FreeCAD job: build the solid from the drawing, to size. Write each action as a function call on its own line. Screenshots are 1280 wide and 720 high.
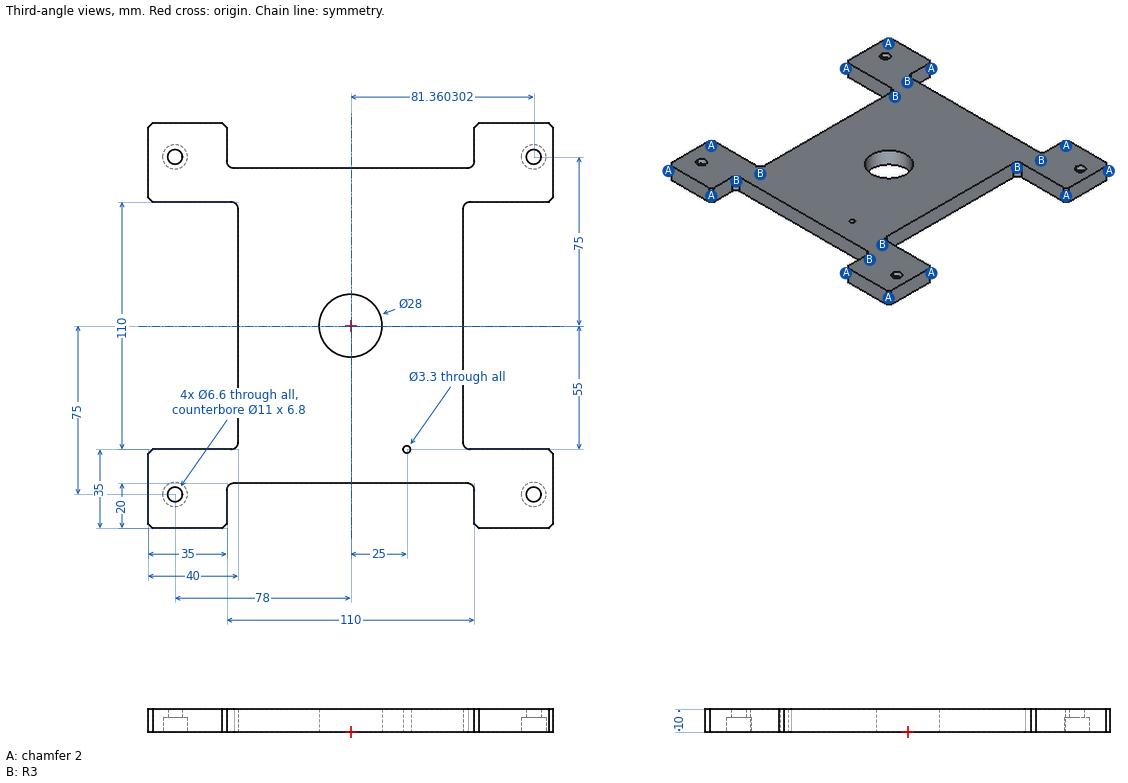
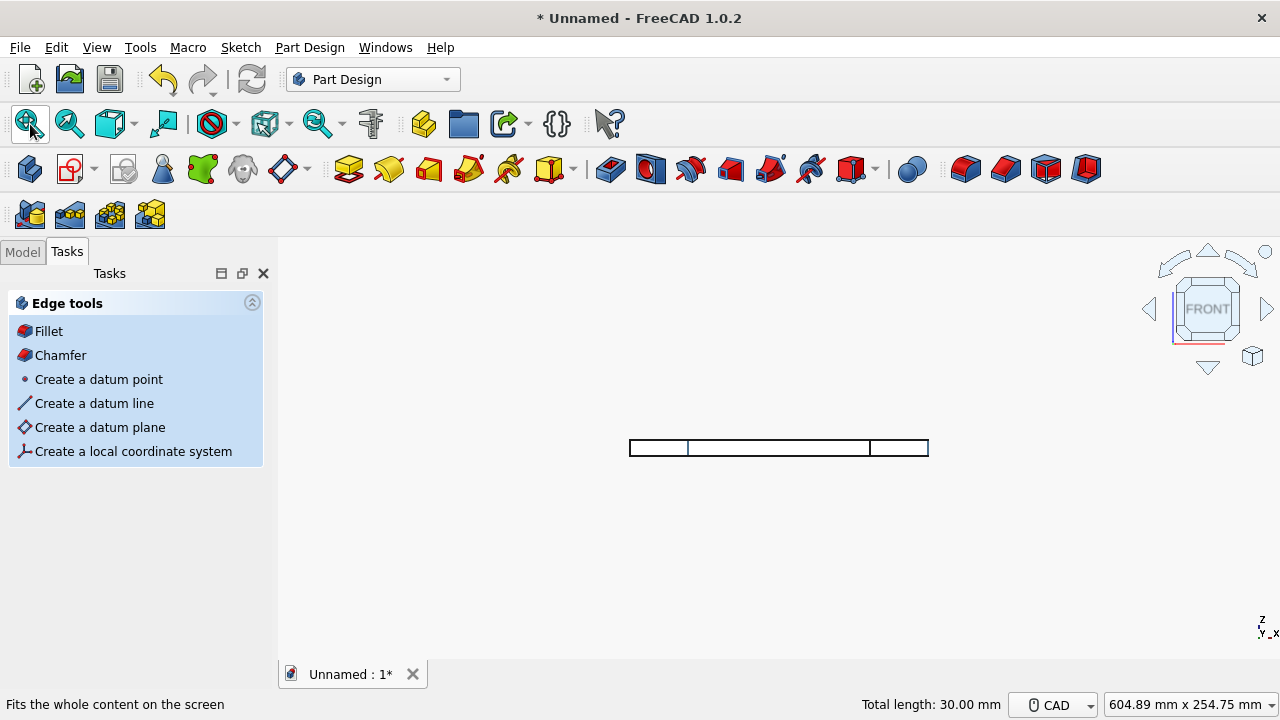
click(870, 447, ctrl)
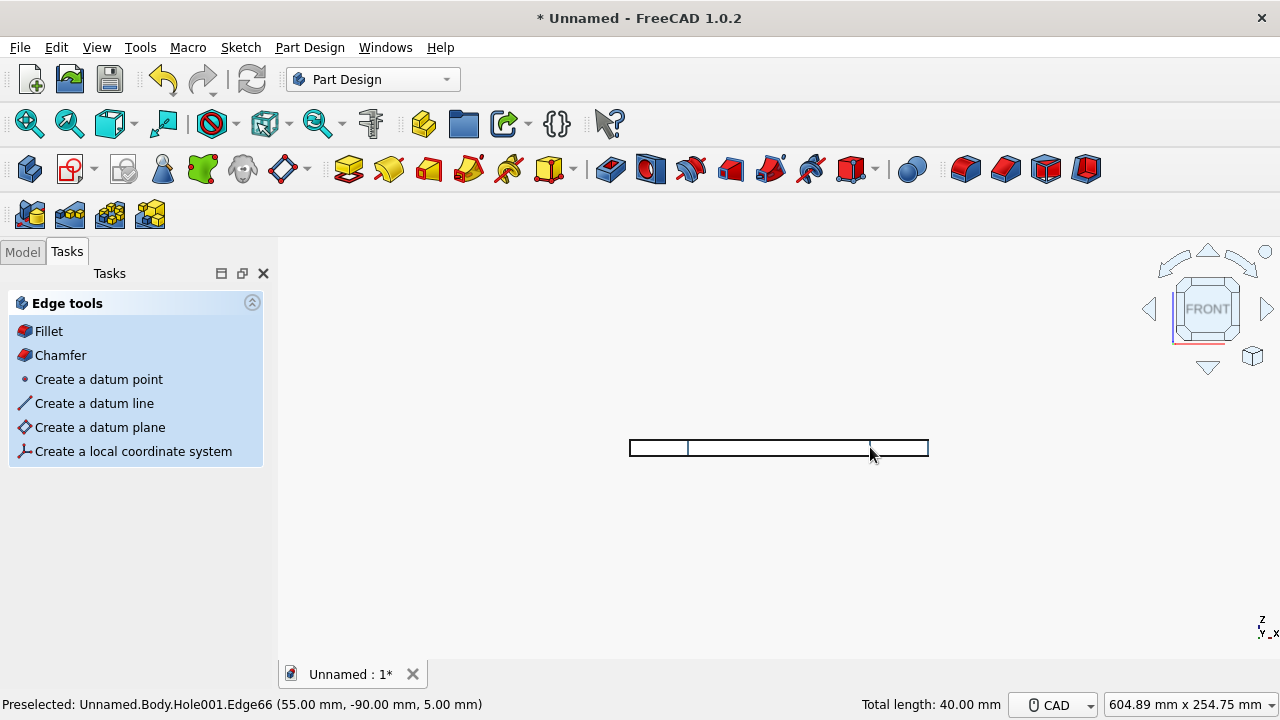
click(630, 447, ctrl)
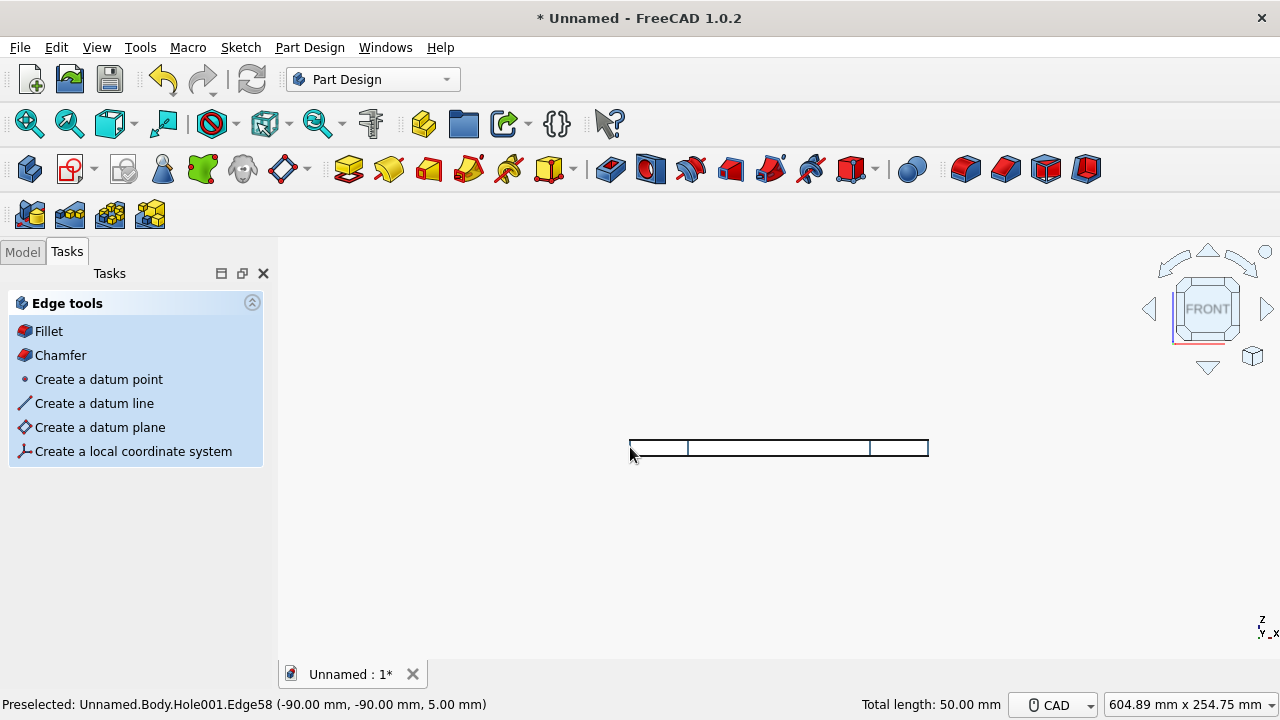
scroll(630, 447, up, 5)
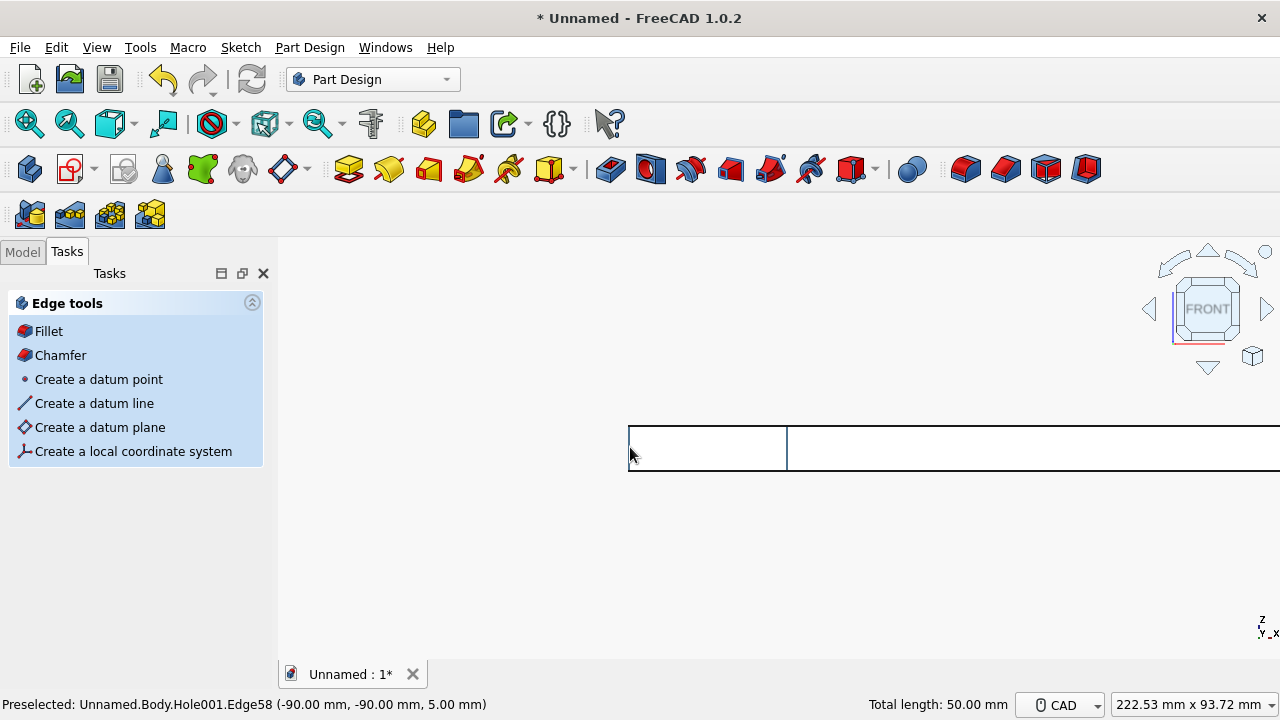
click(30, 124)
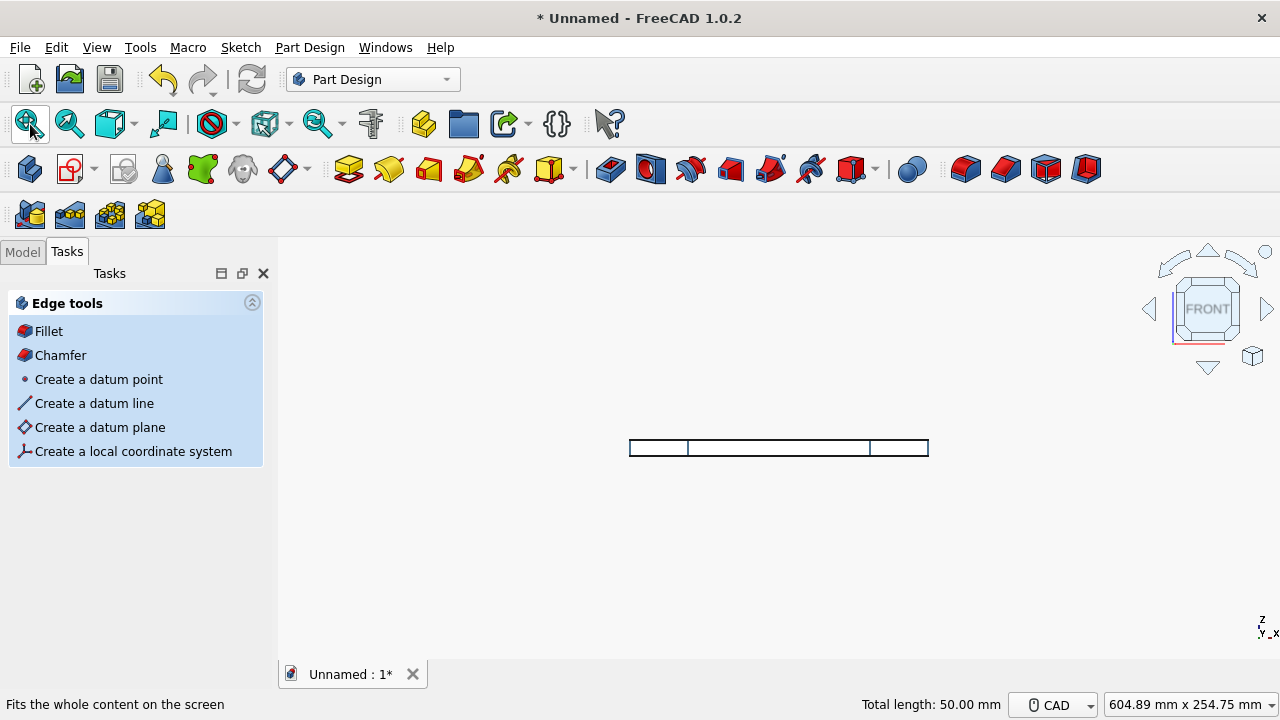
key(3)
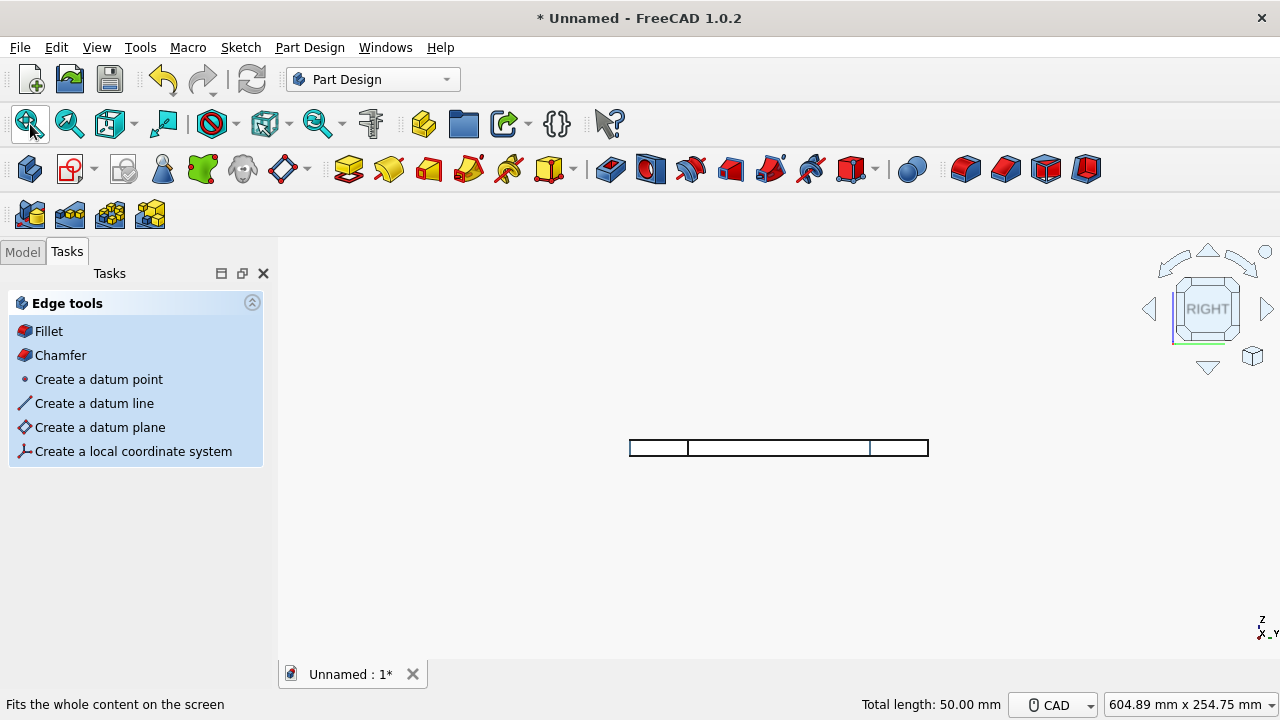
click(30, 124)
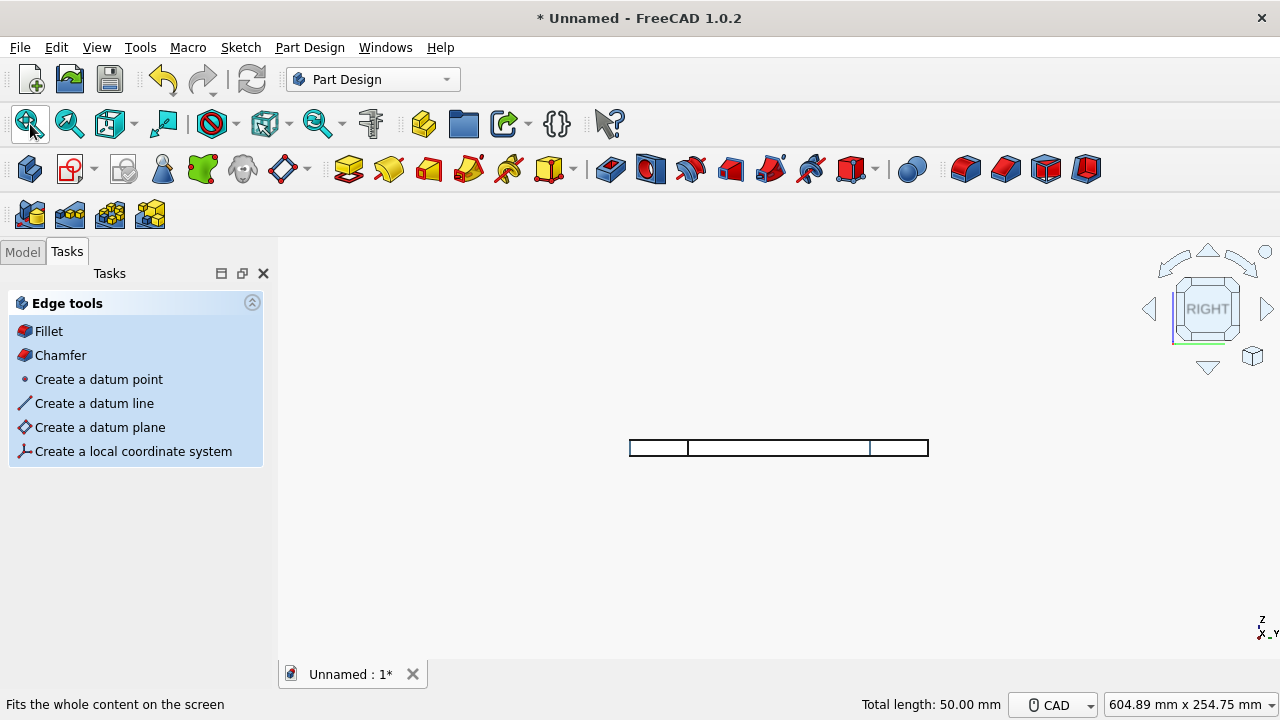
click(928, 447, ctrl)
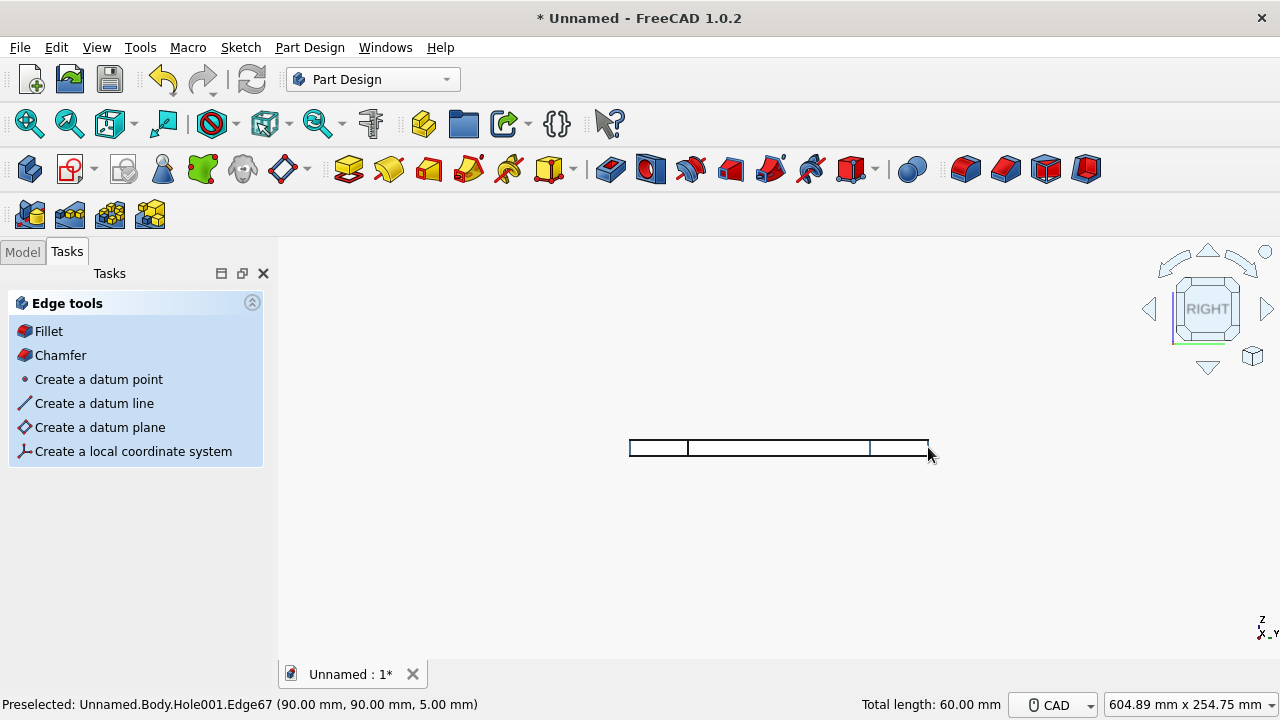
click(688, 447, ctrl)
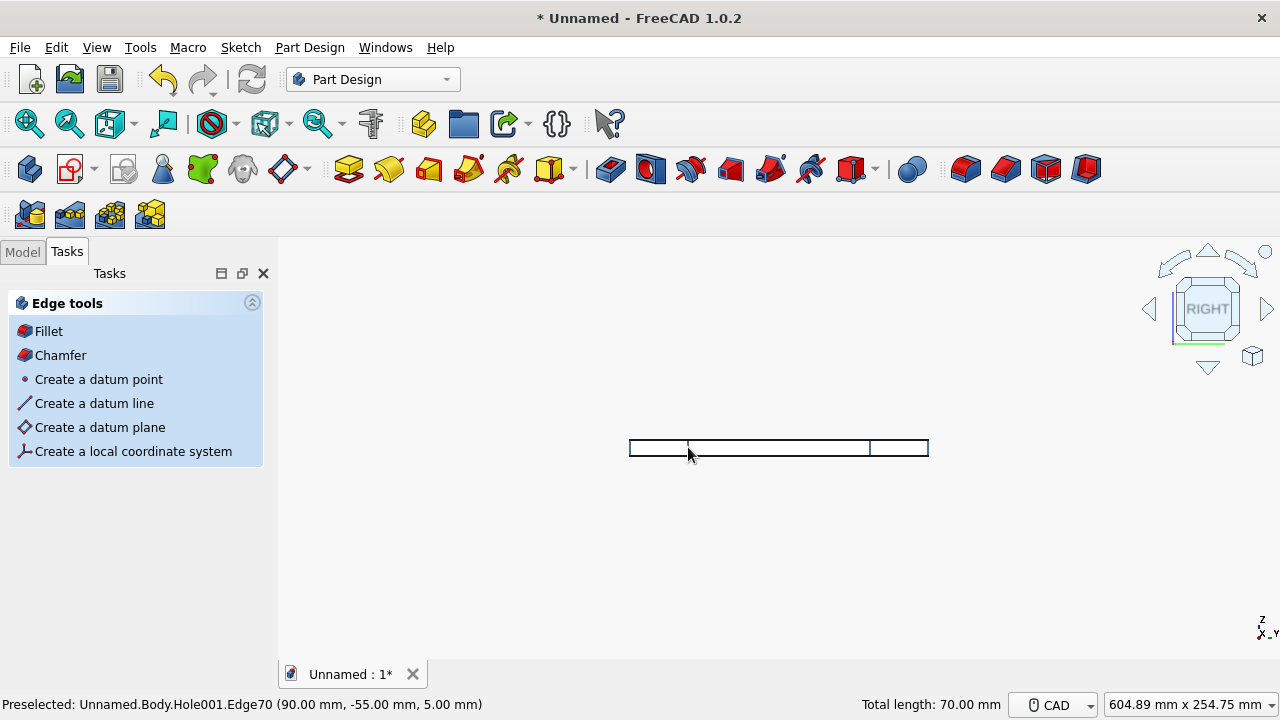
scroll(870, 447, up, 5)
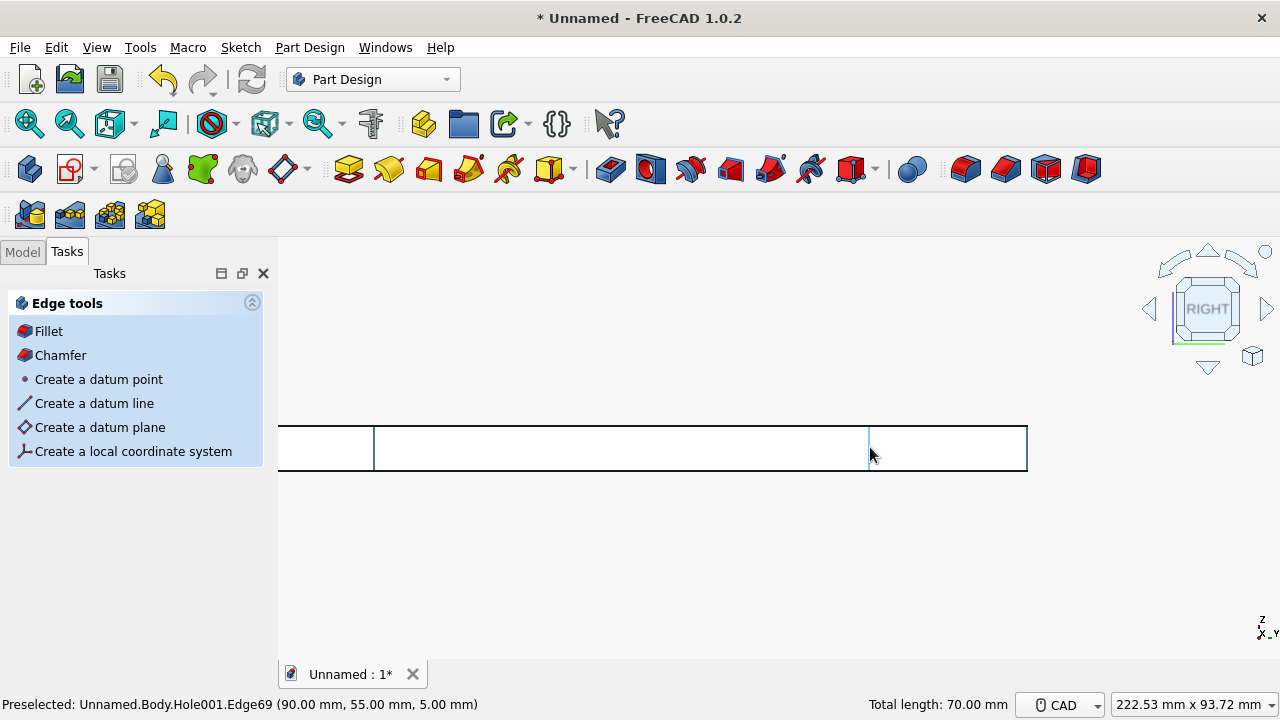
key(v)
key(f)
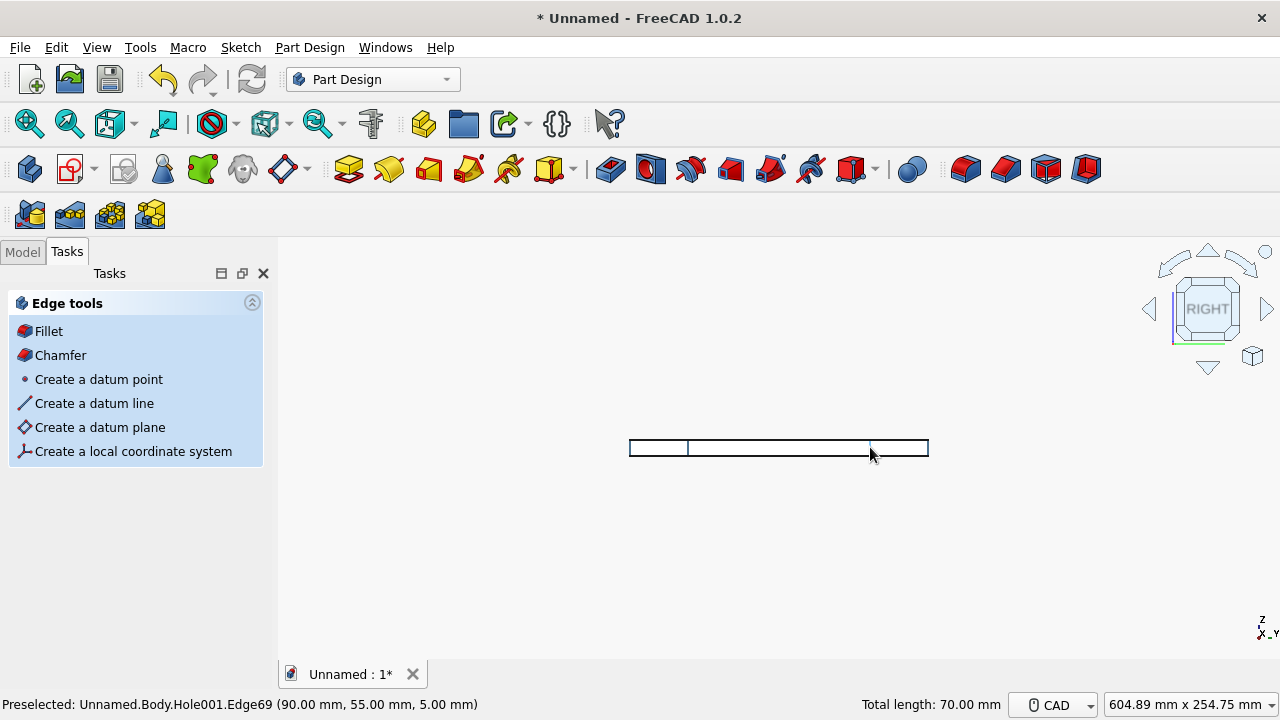
key(5)